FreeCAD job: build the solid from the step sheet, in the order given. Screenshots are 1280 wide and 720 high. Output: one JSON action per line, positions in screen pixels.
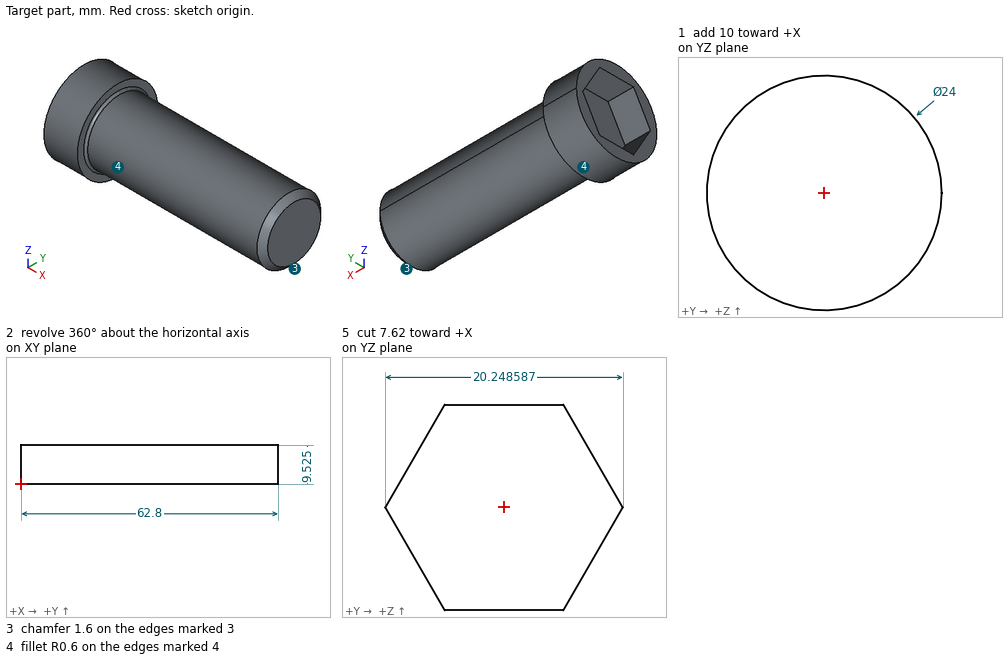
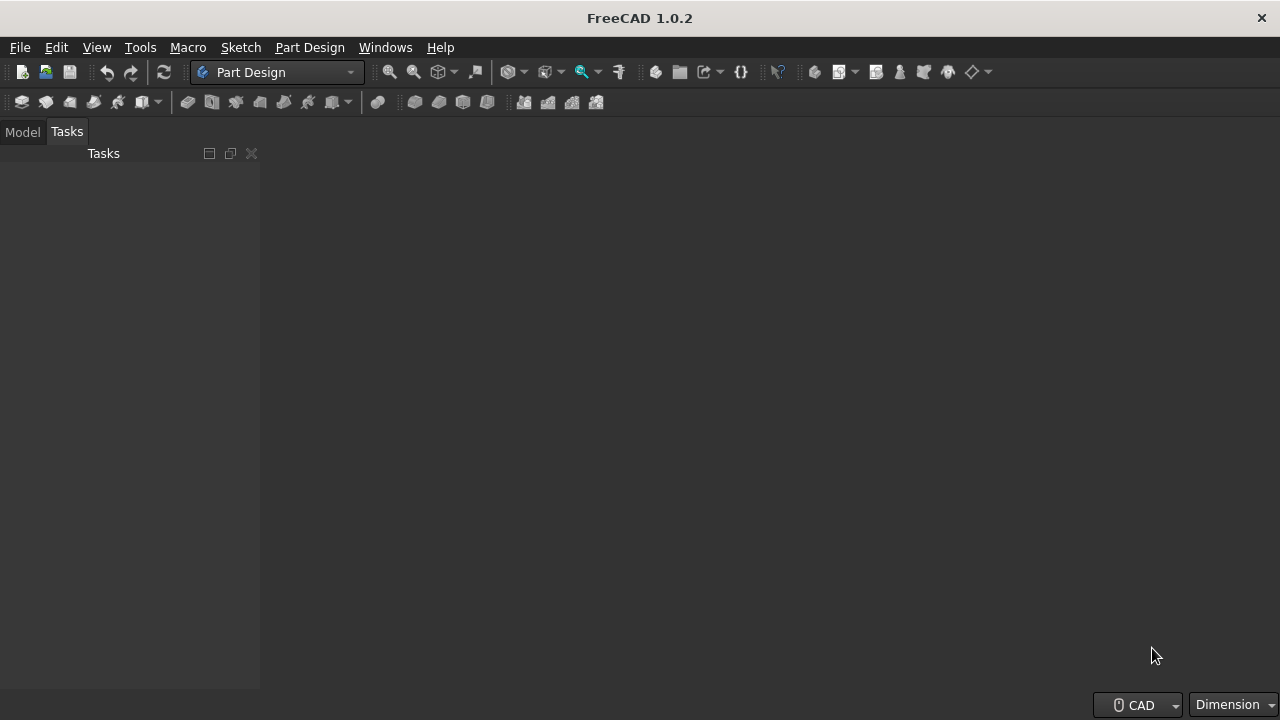
{"action": "left_click", "coordinate": [22, 72]}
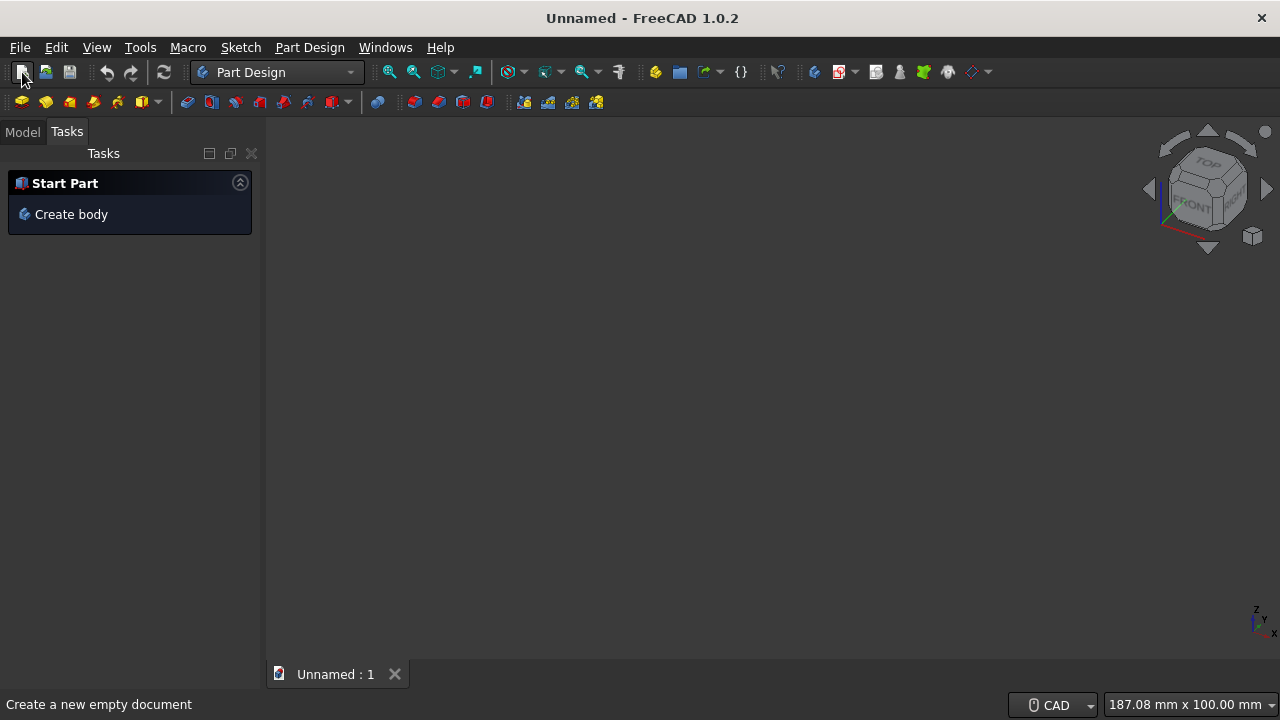
{"action": "left_click", "coordinate": [840, 72]}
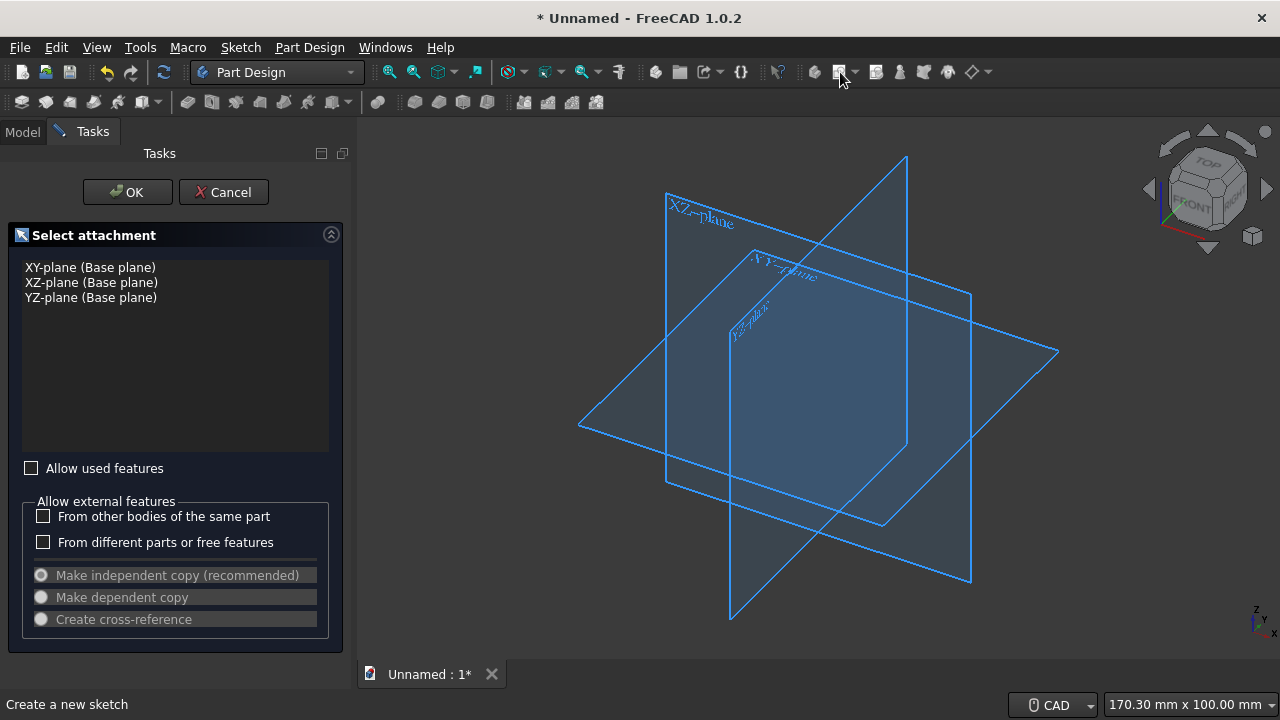
{"action": "left_click", "coordinate": [82, 298]}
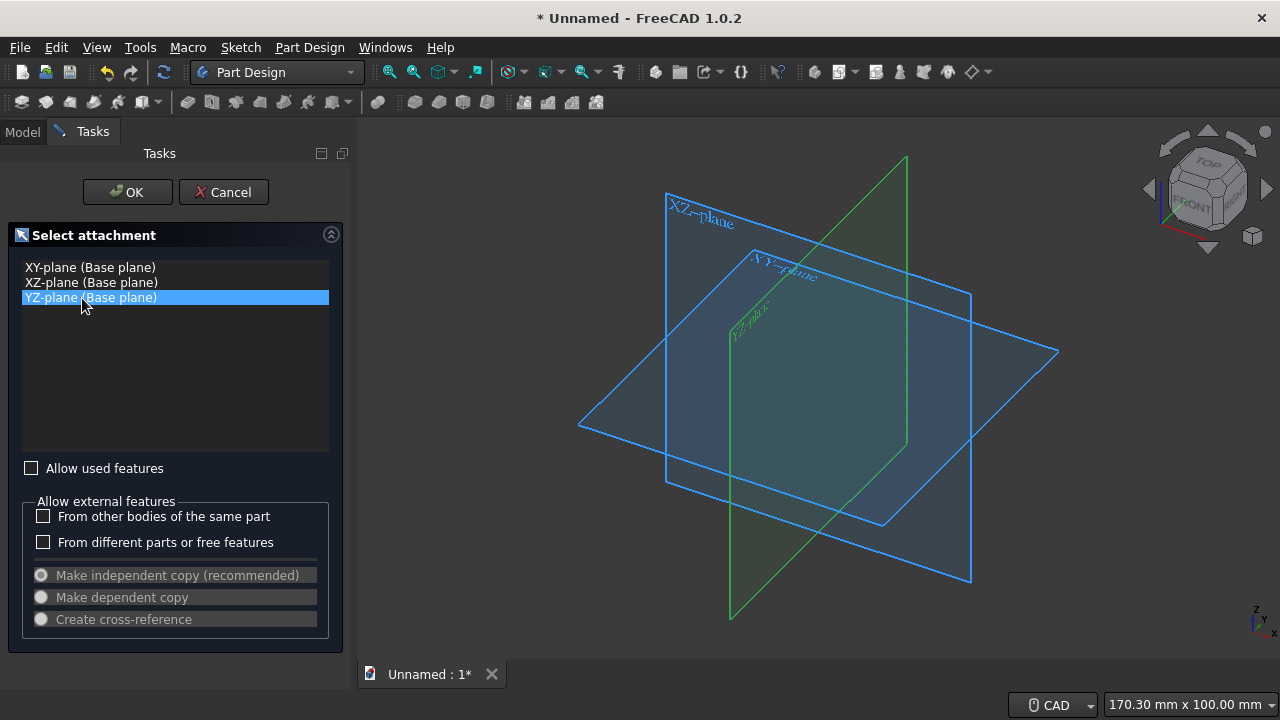
{"action": "left_click", "coordinate": [128, 192]}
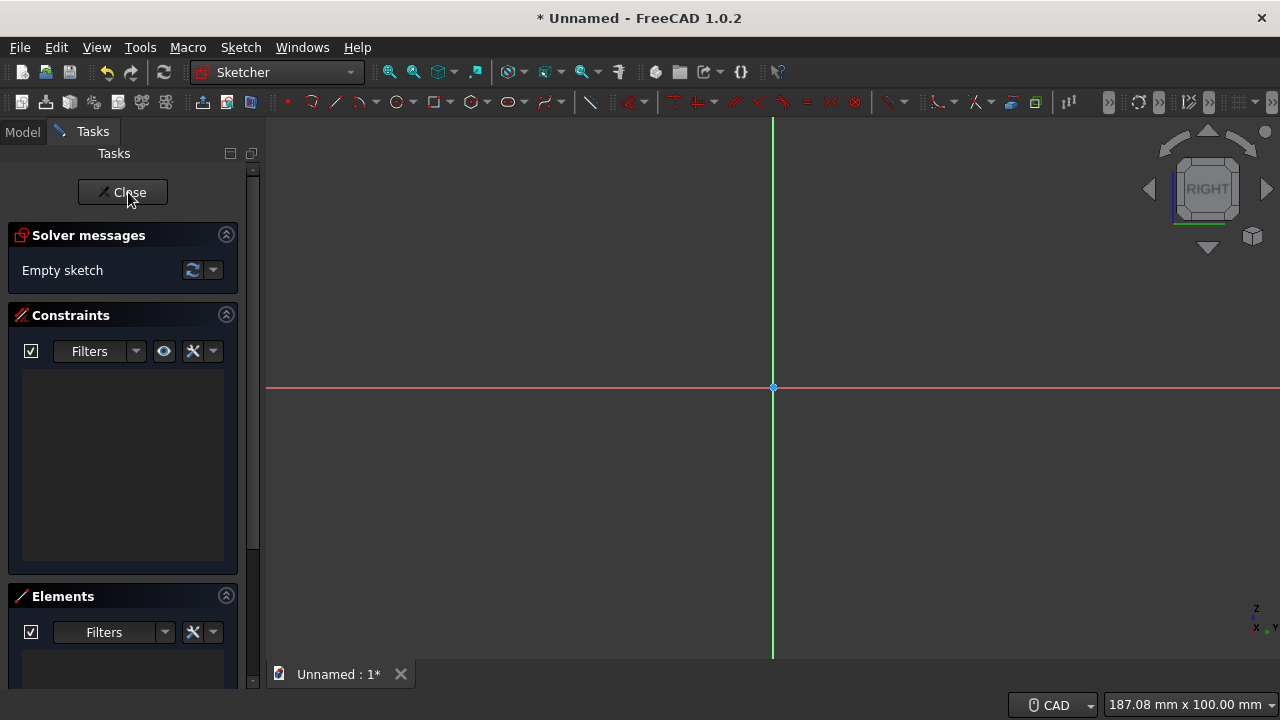
{"action": "scroll", "coordinate": [813, 388], "scroll_direction": "up", "scroll_amount": 5}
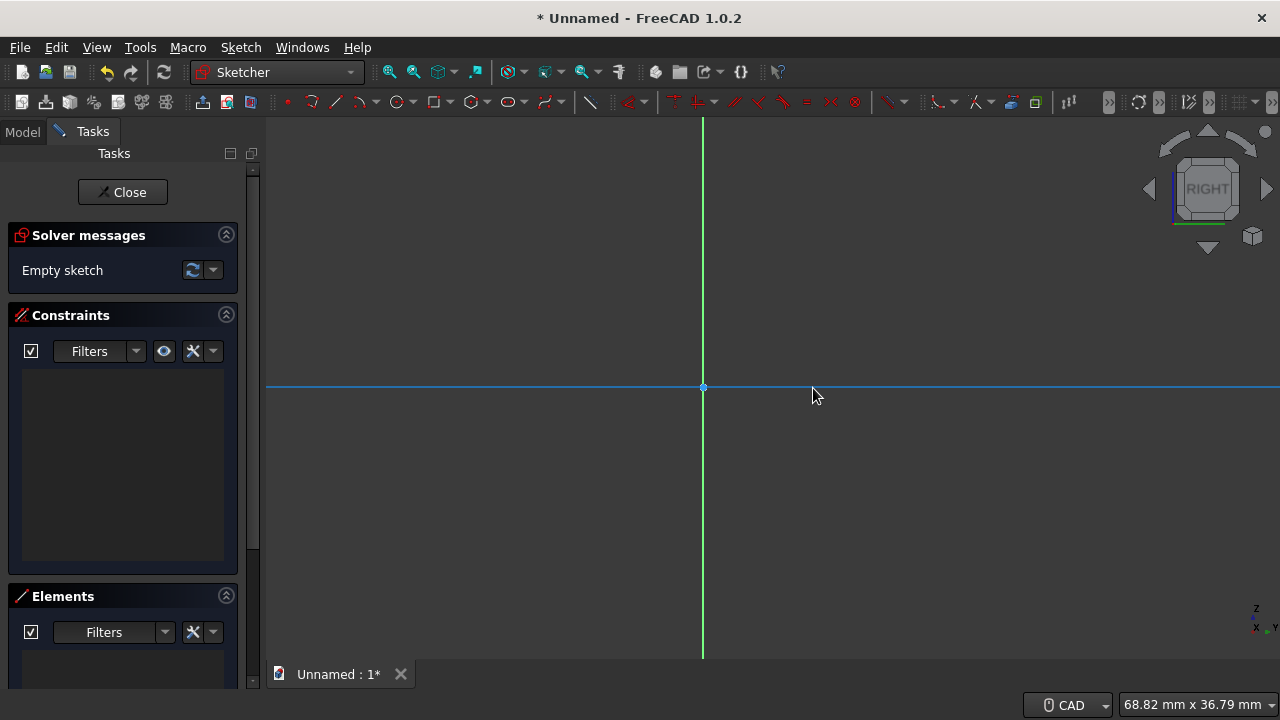
{"action": "left_click", "coordinate": [398, 102]}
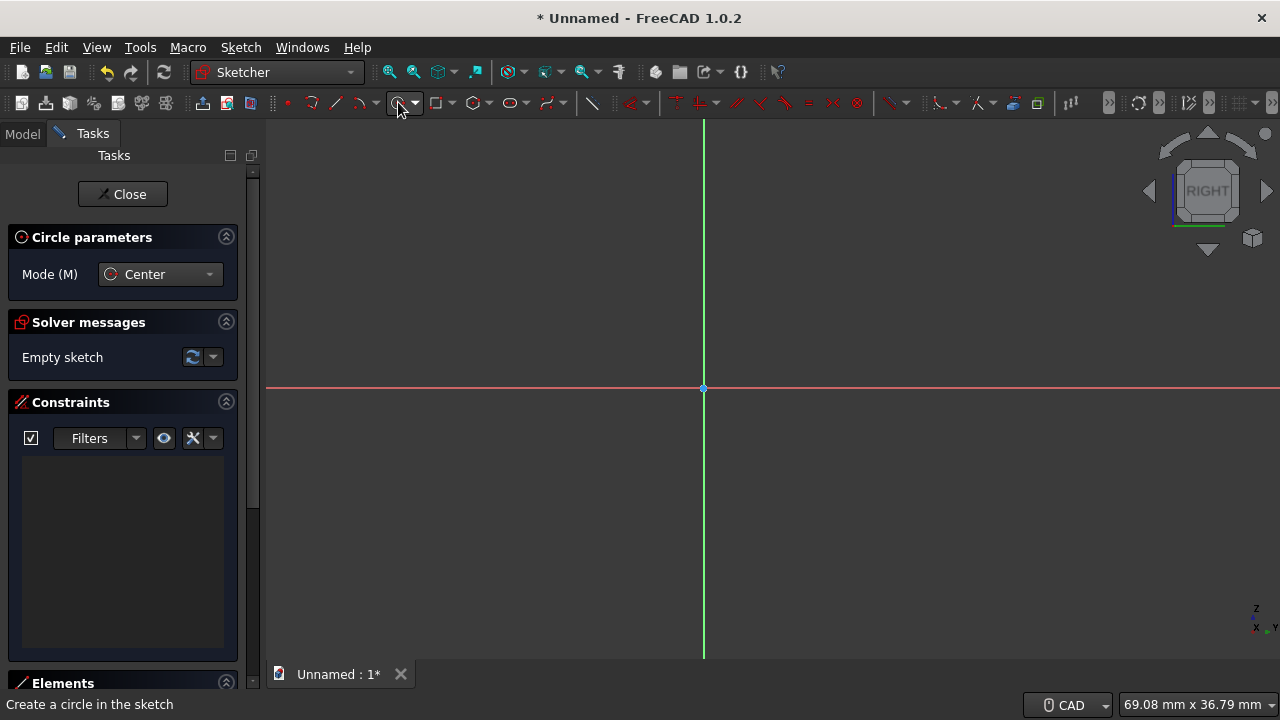
{"action": "left_click", "coordinate": [704, 388]}
{"action": "left_click", "coordinate": [828, 264]}
{"action": "key", "text": "Escape"}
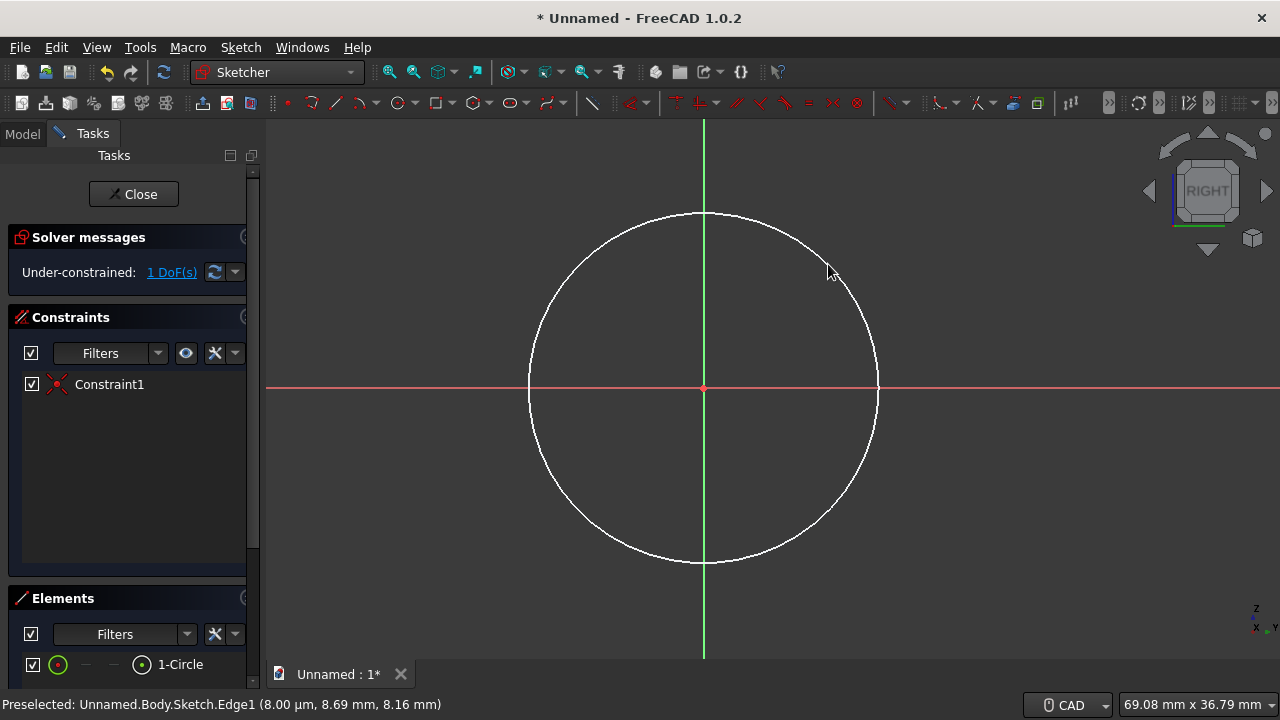
{"action": "left_click", "coordinate": [827, 264]}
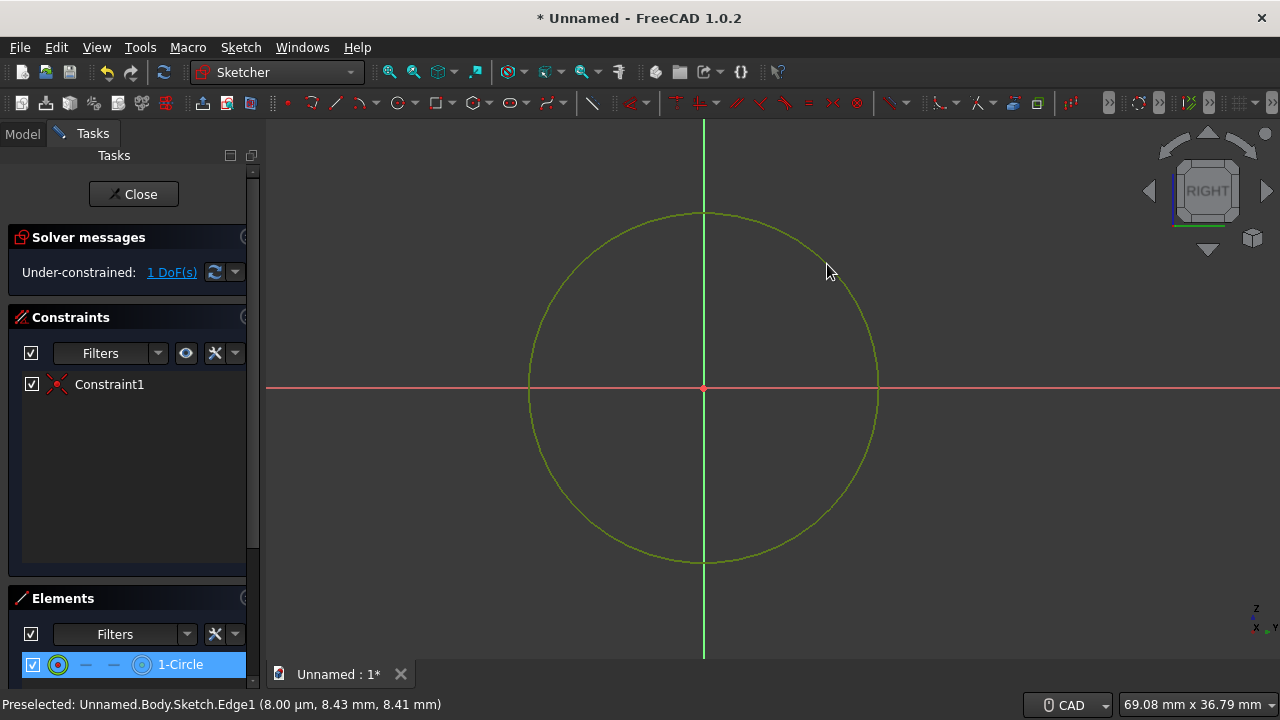
{"action": "key", "text": "k o"}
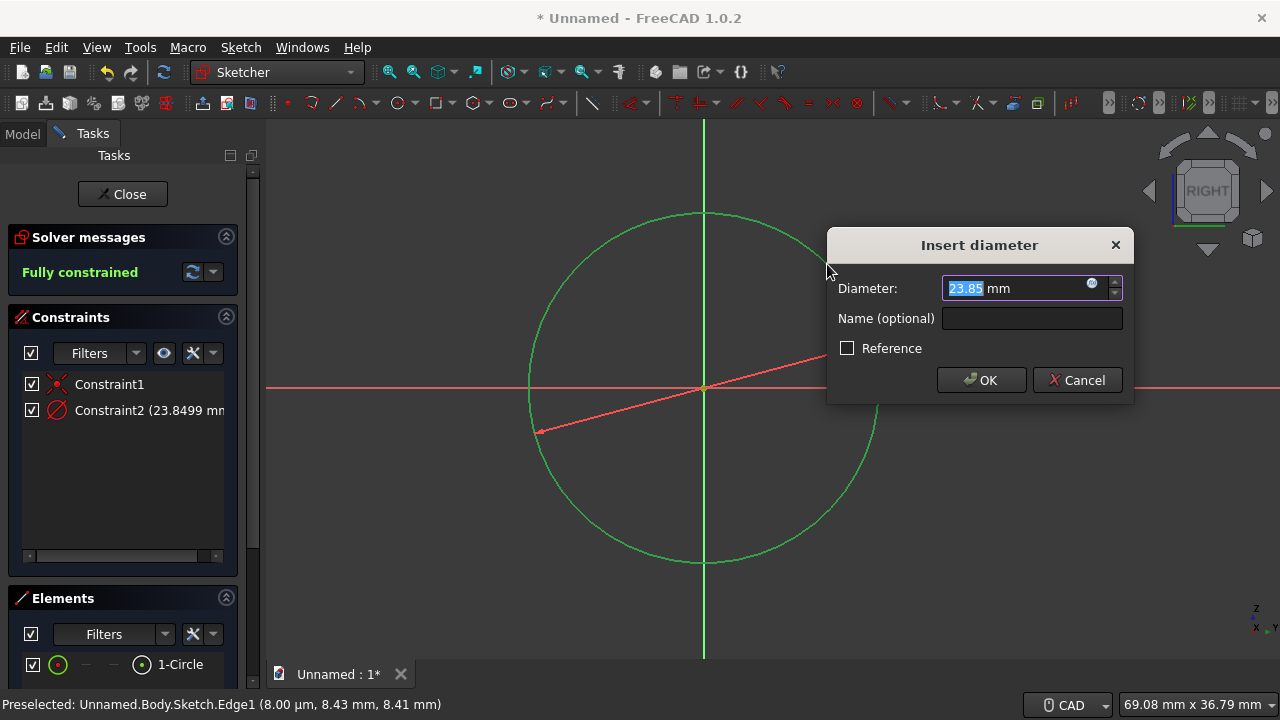
{"action": "type", "text": "24"}
{"action": "key", "text": "Return"}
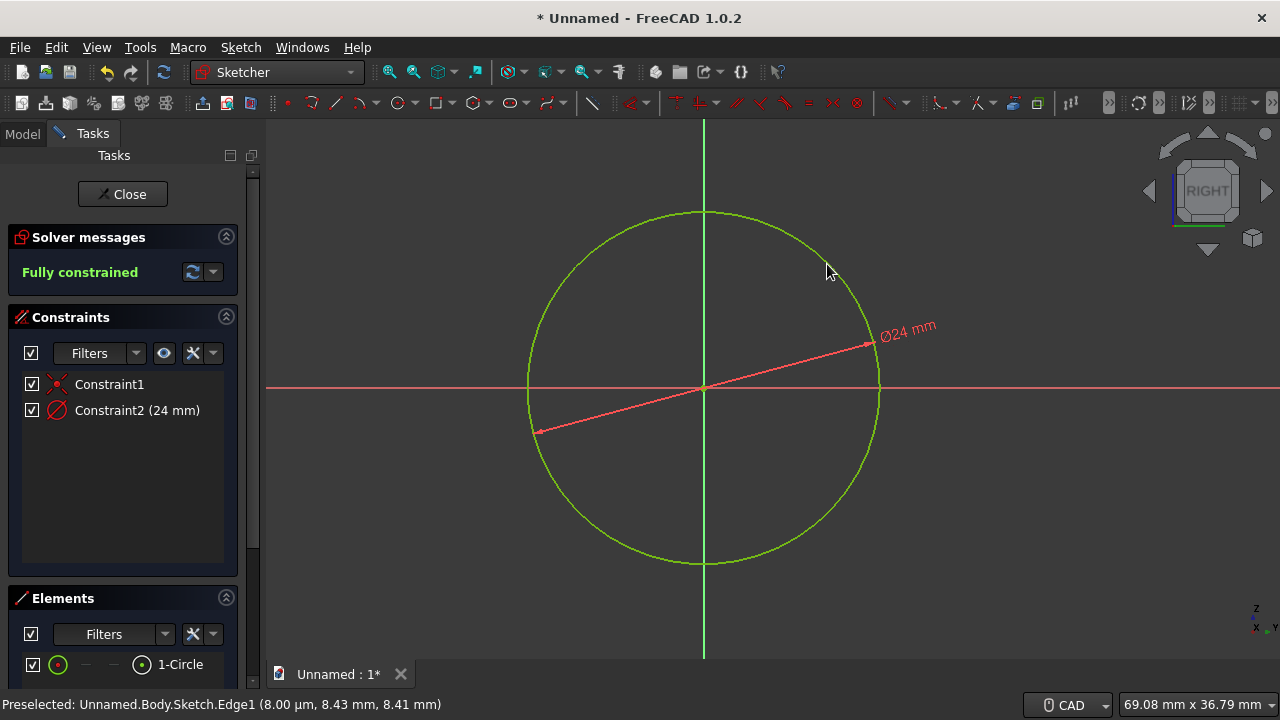
{"action": "left_click", "coordinate": [123, 194]}